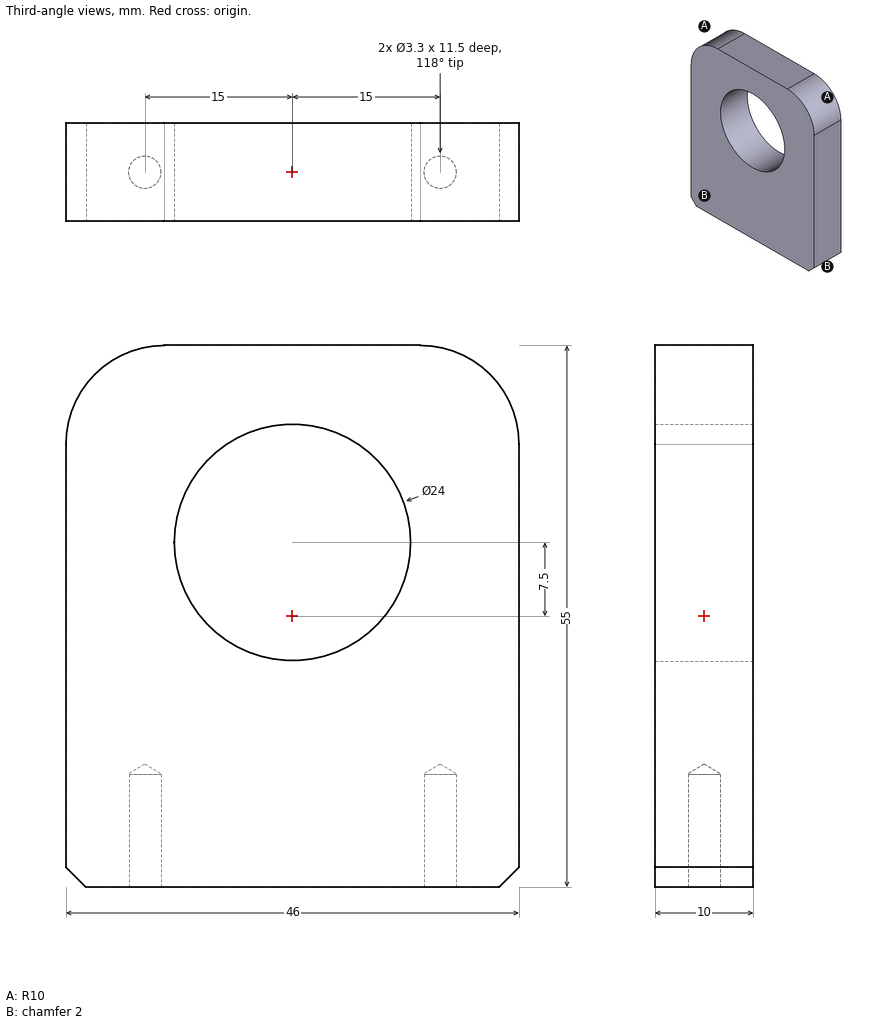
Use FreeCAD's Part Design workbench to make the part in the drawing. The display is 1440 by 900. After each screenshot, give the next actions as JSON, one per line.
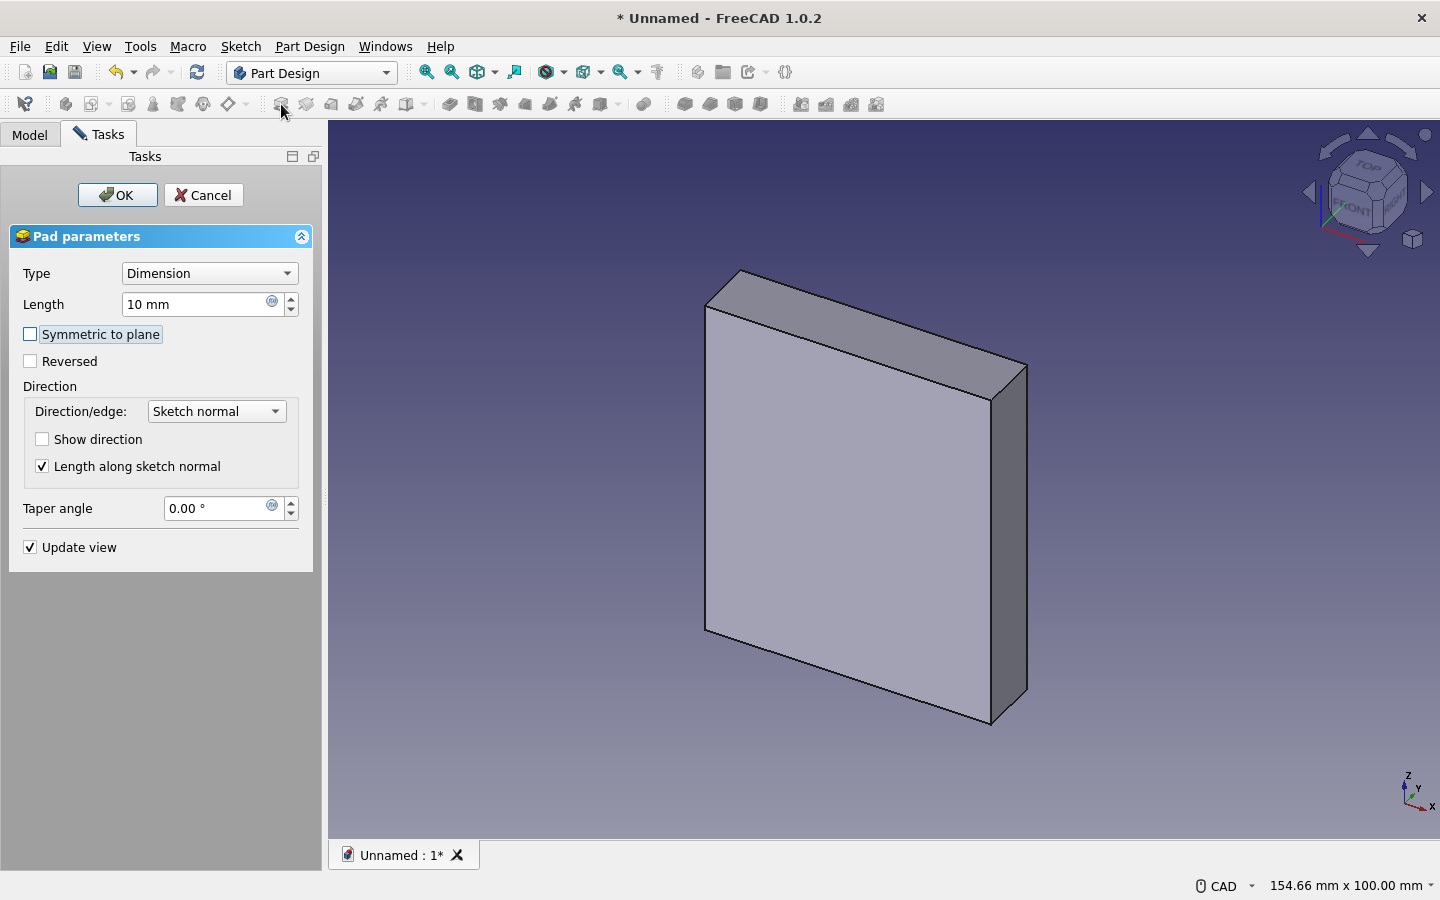
{"action": "left_click", "coordinate": [31, 334]}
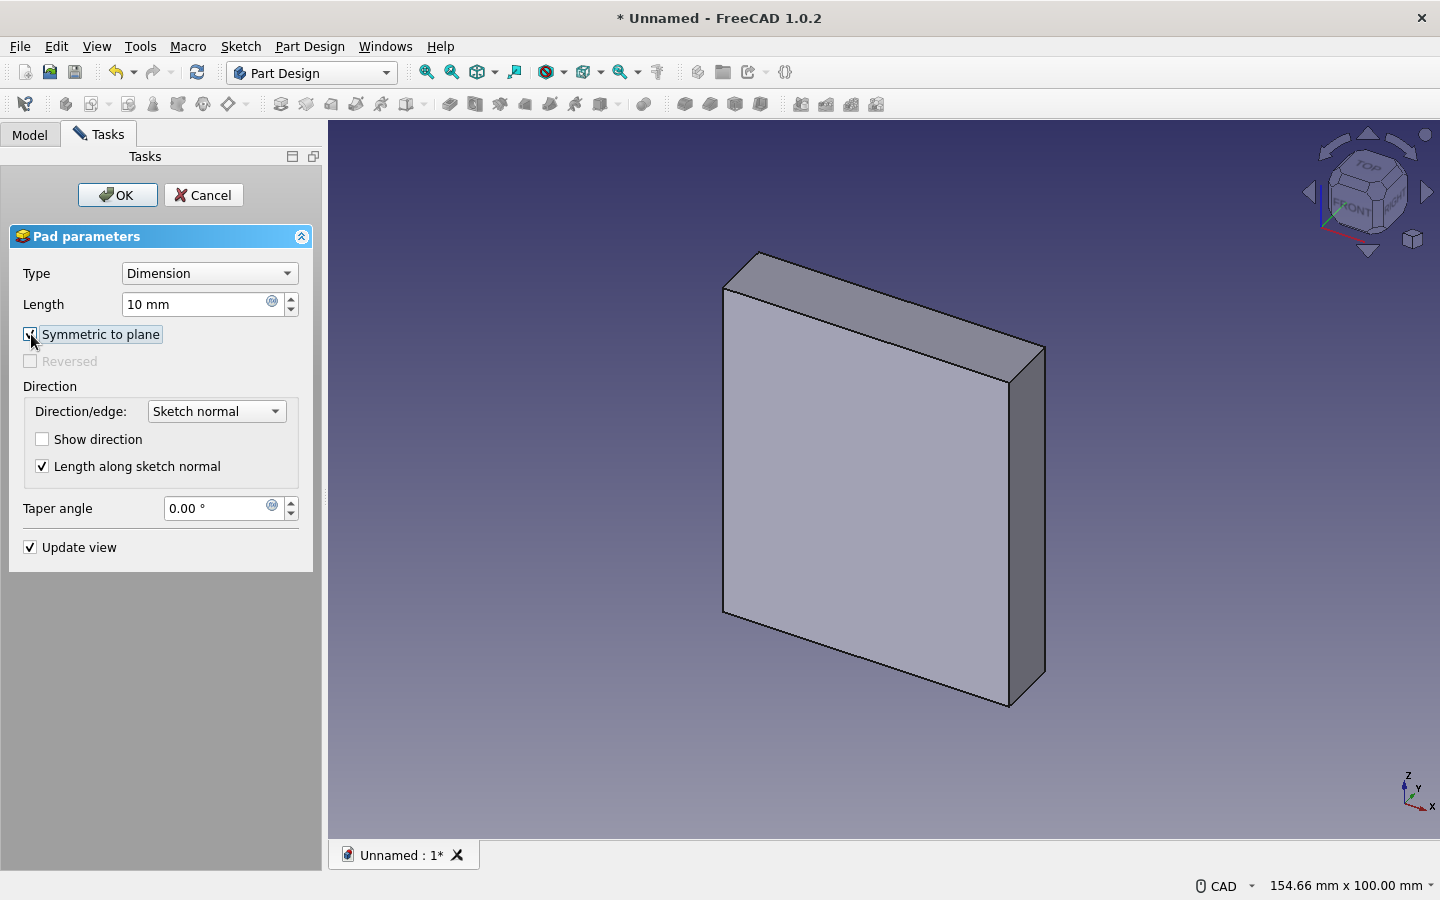
{"action": "left_click", "coordinate": [118, 195]}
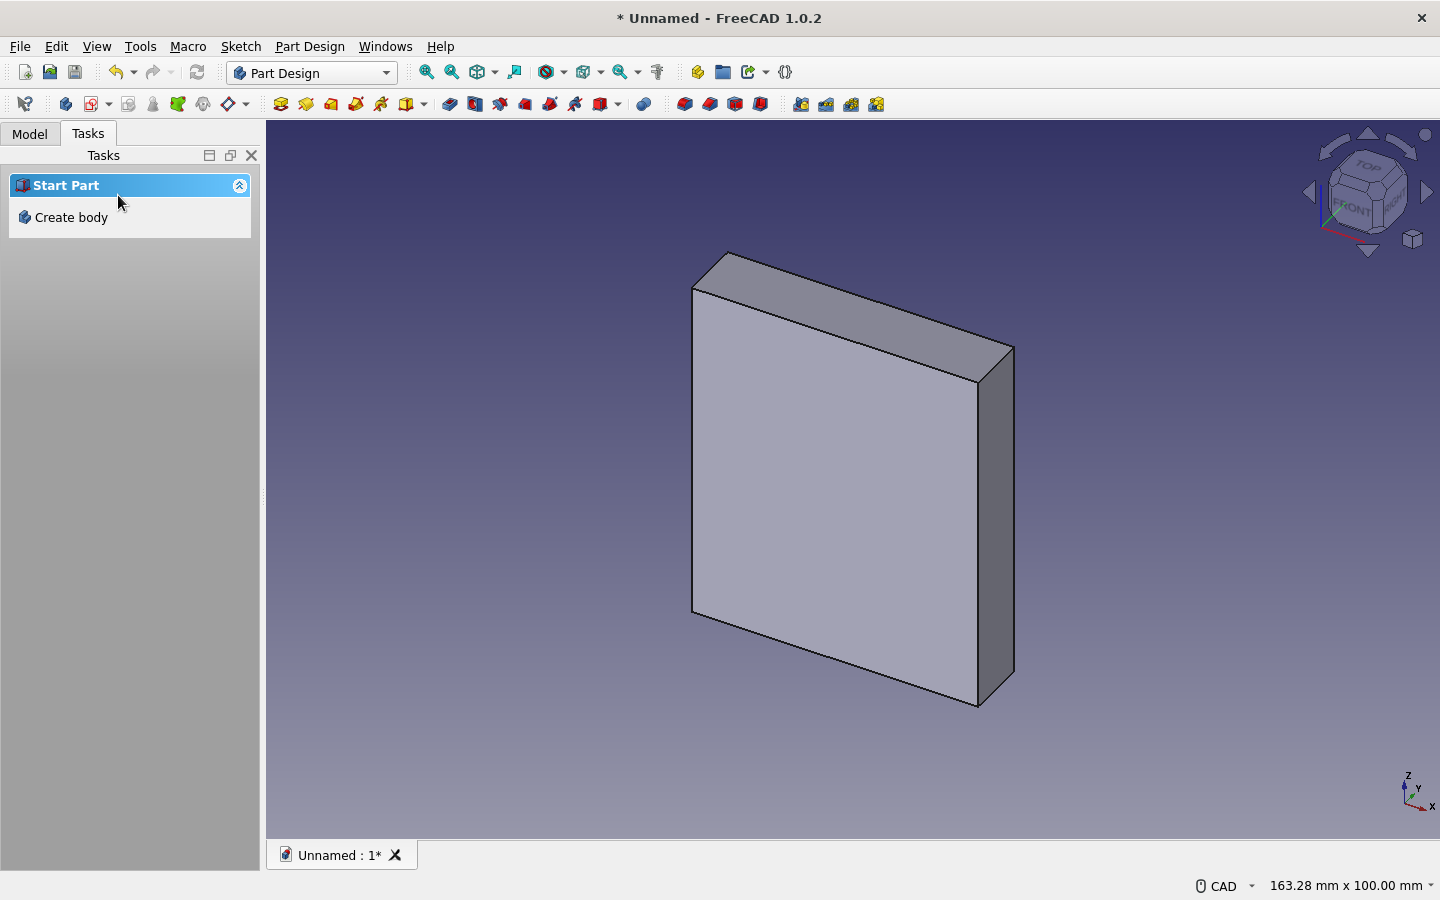
{"action": "key", "text": "4"}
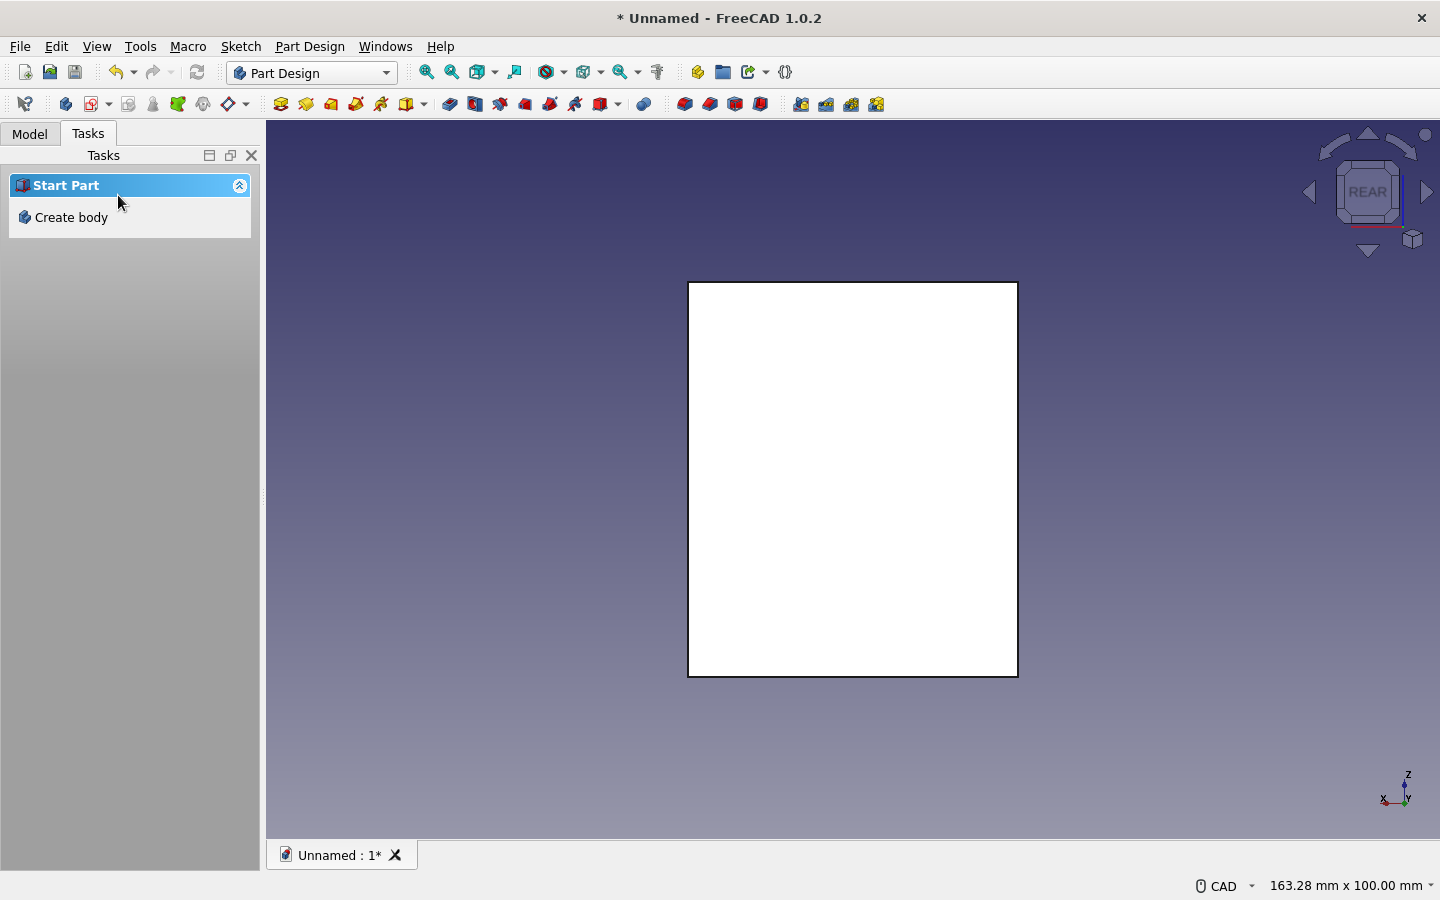
{"action": "left_click", "coordinate": [853, 478]}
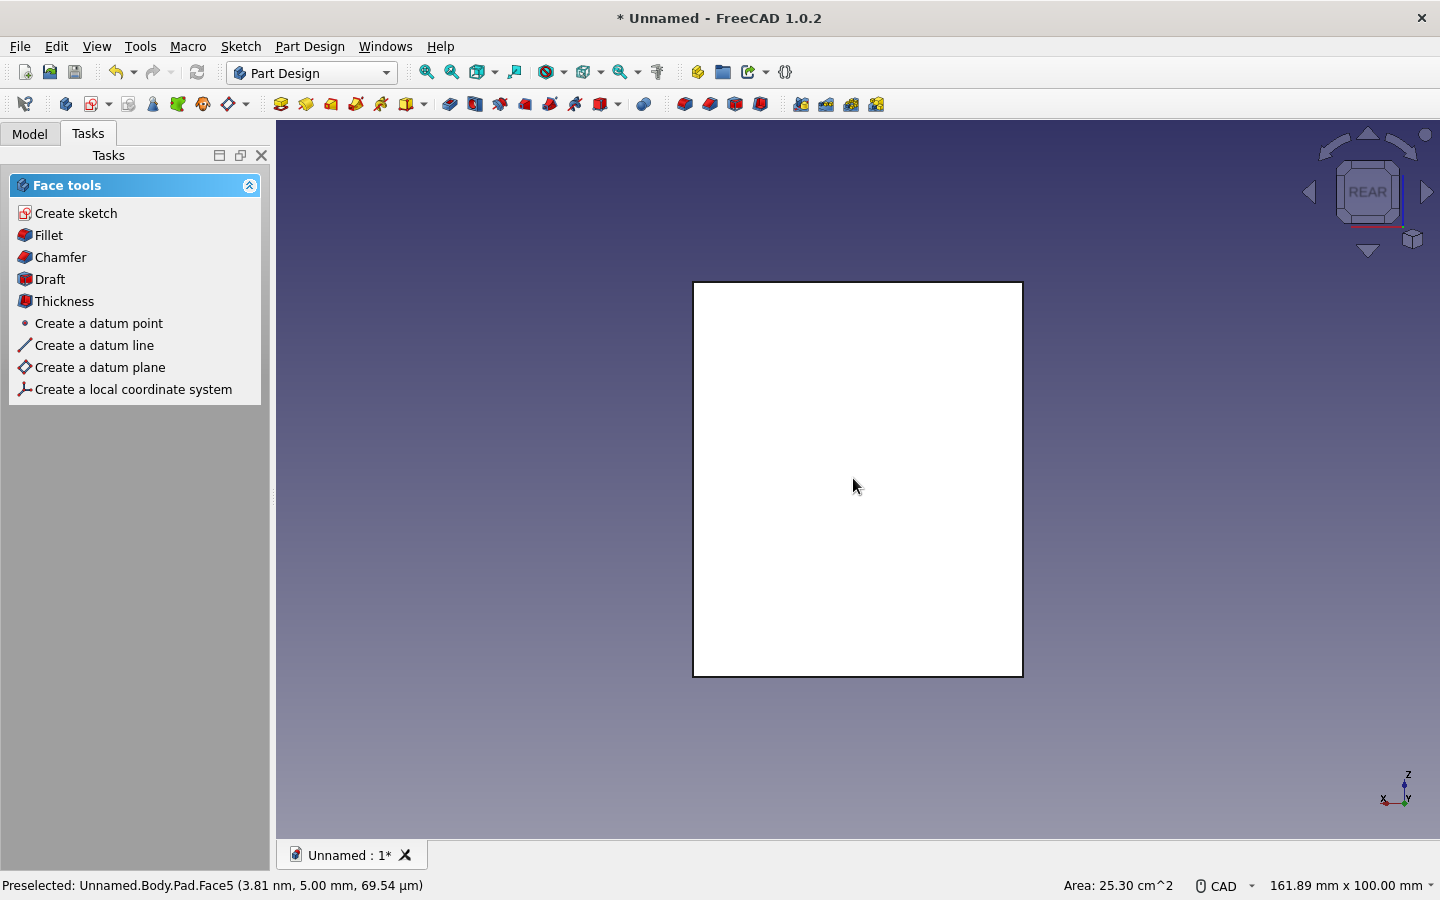
{"action": "left_click", "coordinate": [90, 104]}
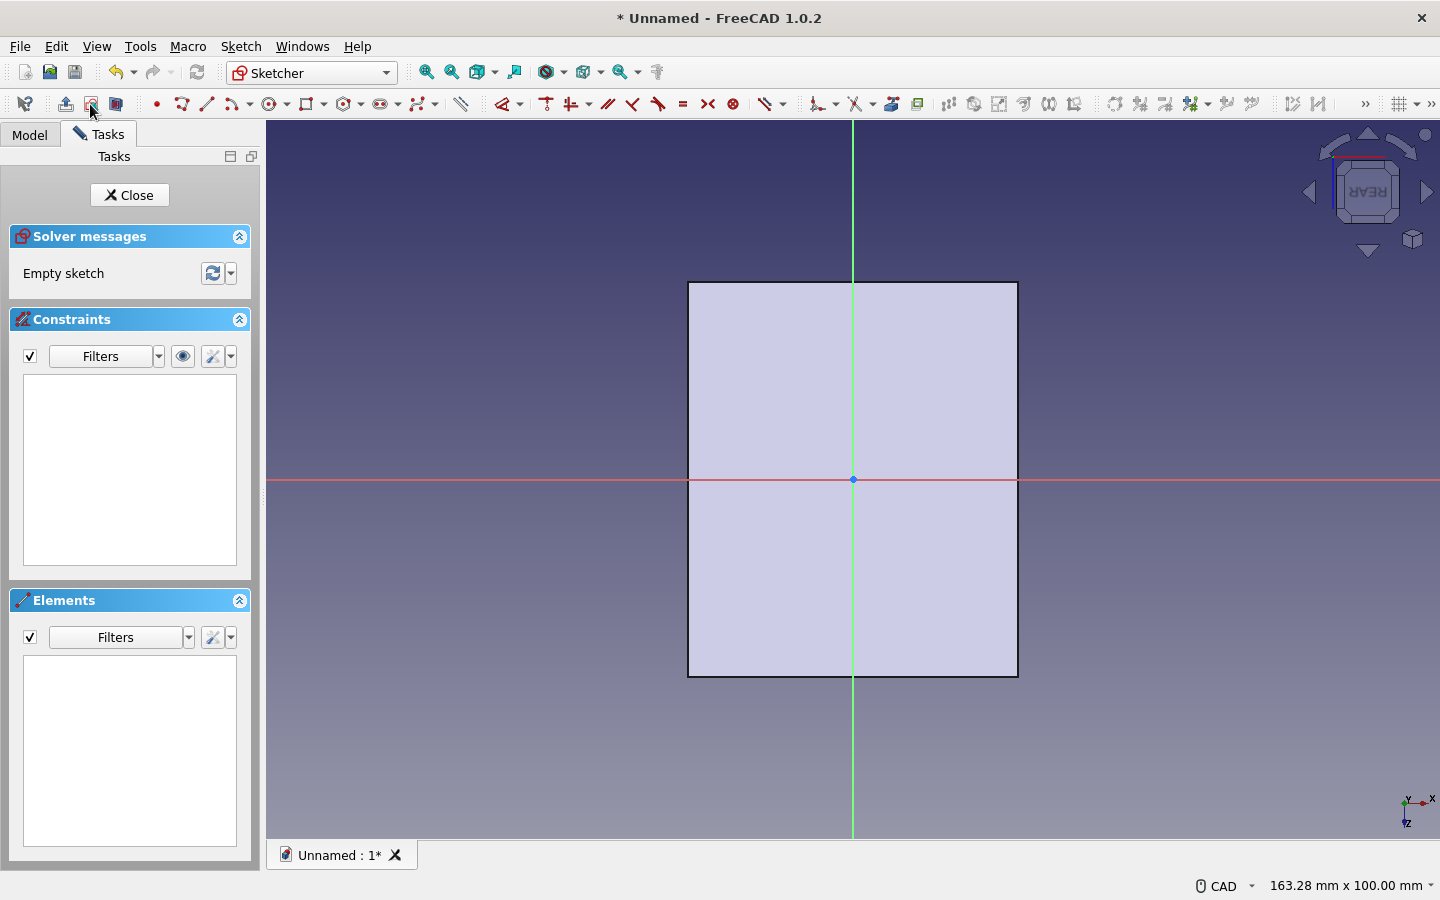
{"action": "scroll", "coordinate": [893, 565], "scroll_direction": "up", "scroll_amount": 5}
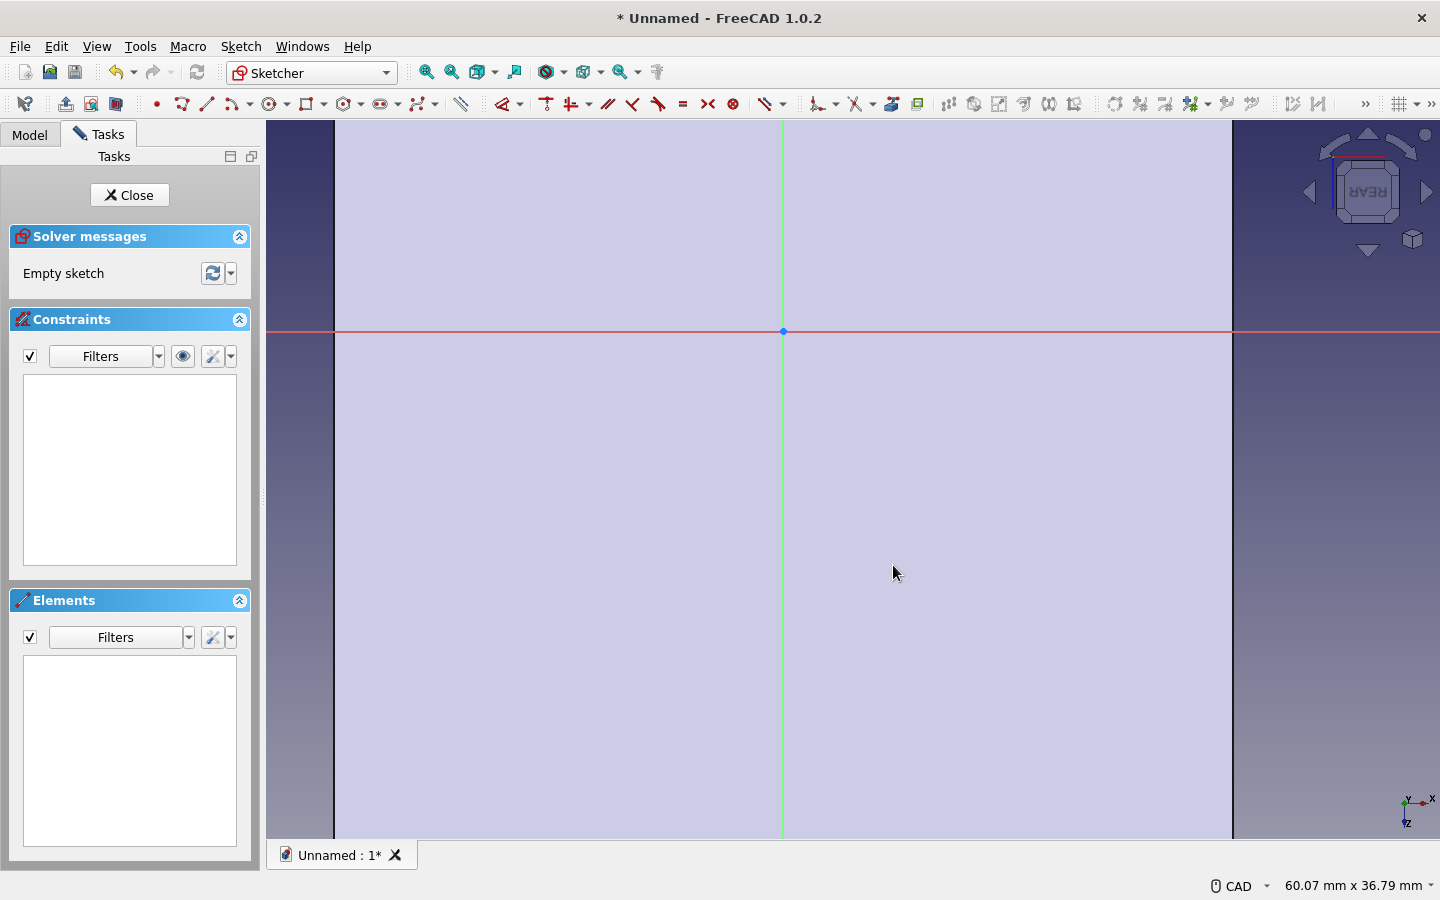
{"action": "left_click", "coordinate": [268, 104]}